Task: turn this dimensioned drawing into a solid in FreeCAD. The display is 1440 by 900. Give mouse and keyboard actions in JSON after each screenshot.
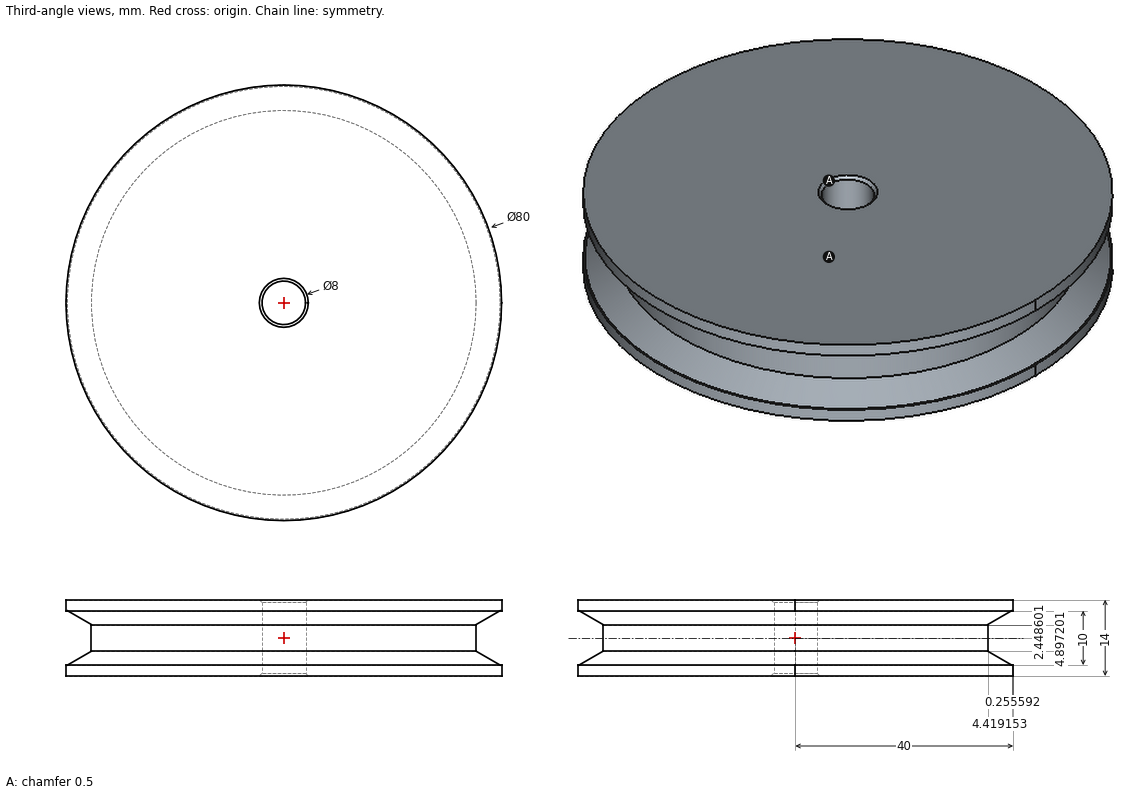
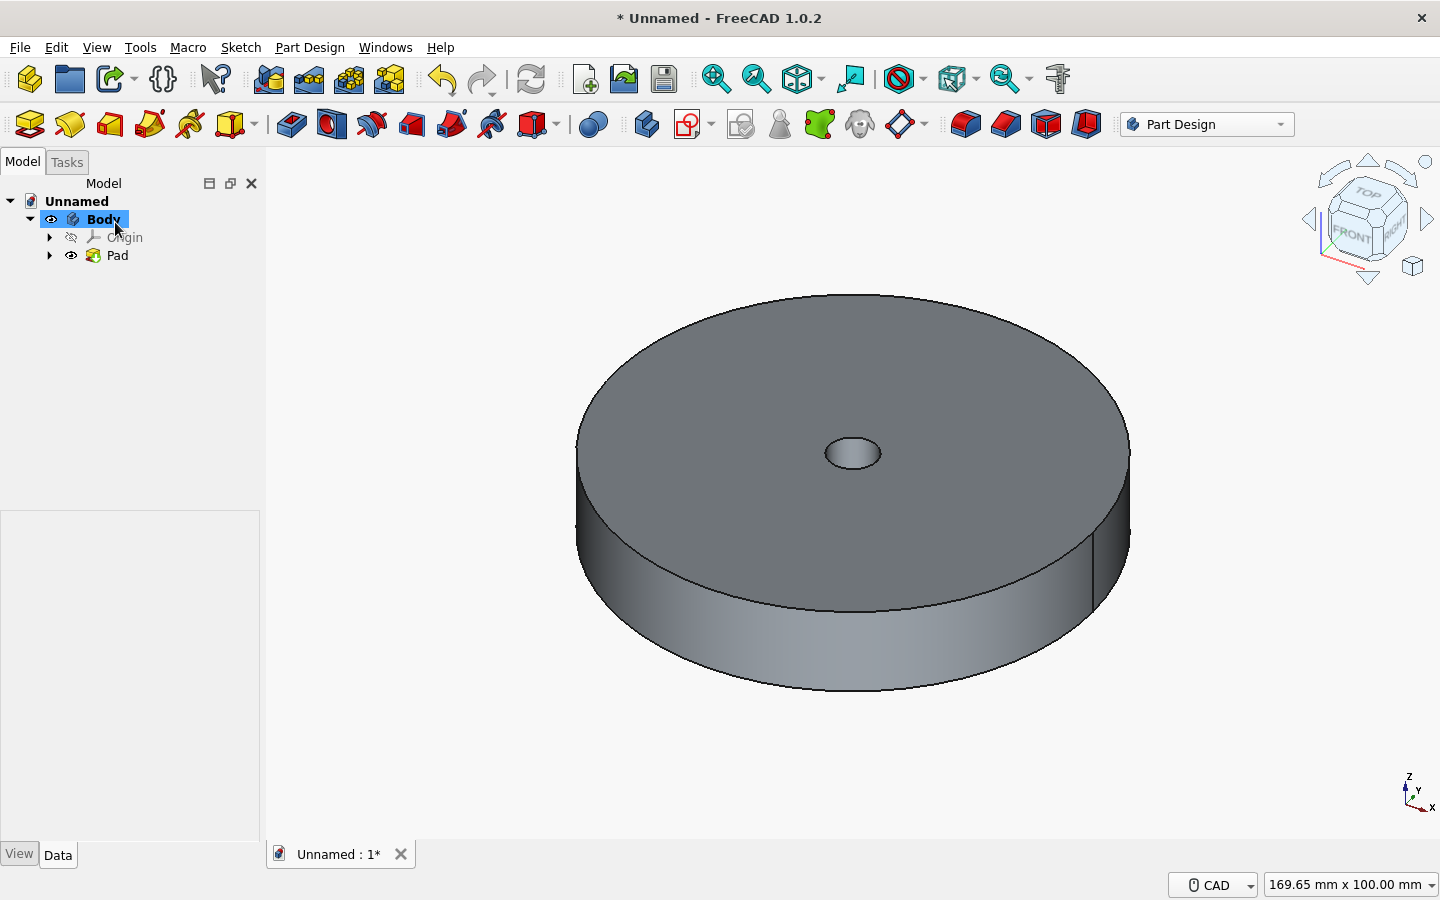
{"action": "left_click", "coordinate": [688, 124]}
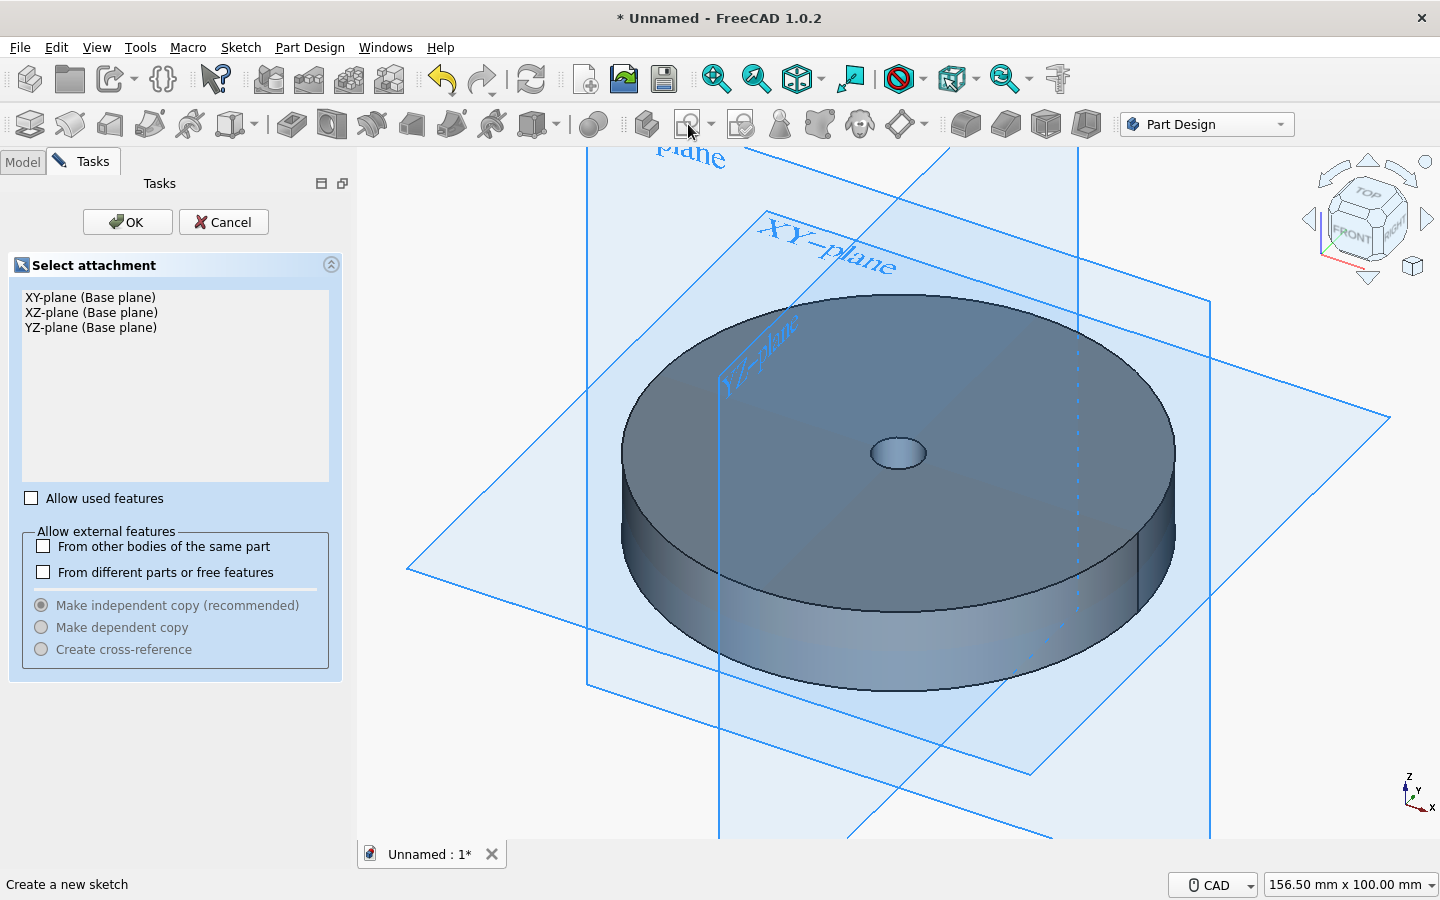
{"action": "left_click", "coordinate": [82, 328]}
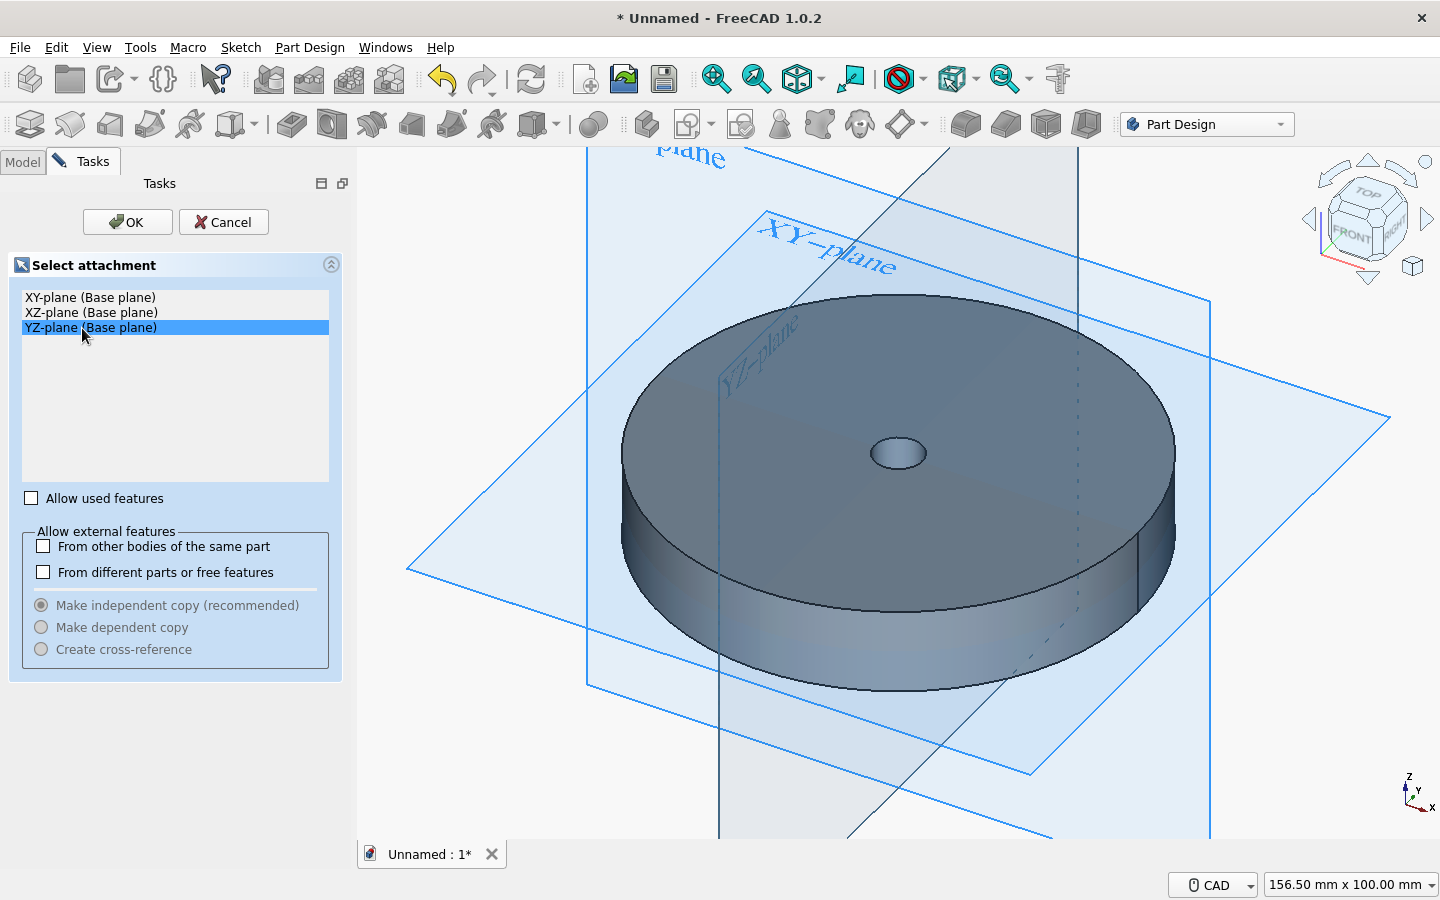
{"action": "left_click", "coordinate": [128, 222]}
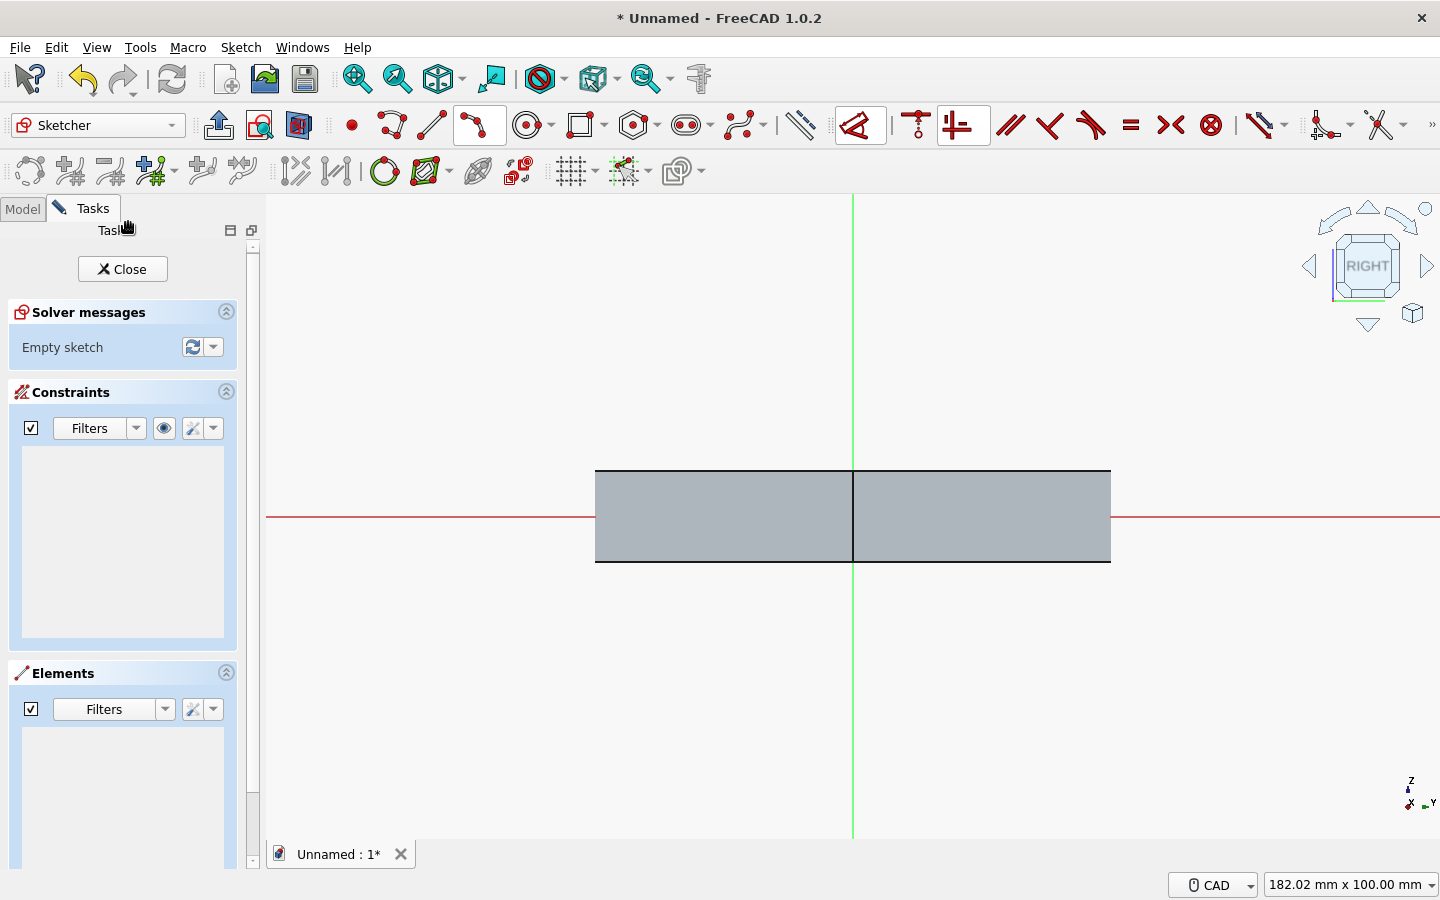
{"action": "left_click", "coordinate": [300, 126]}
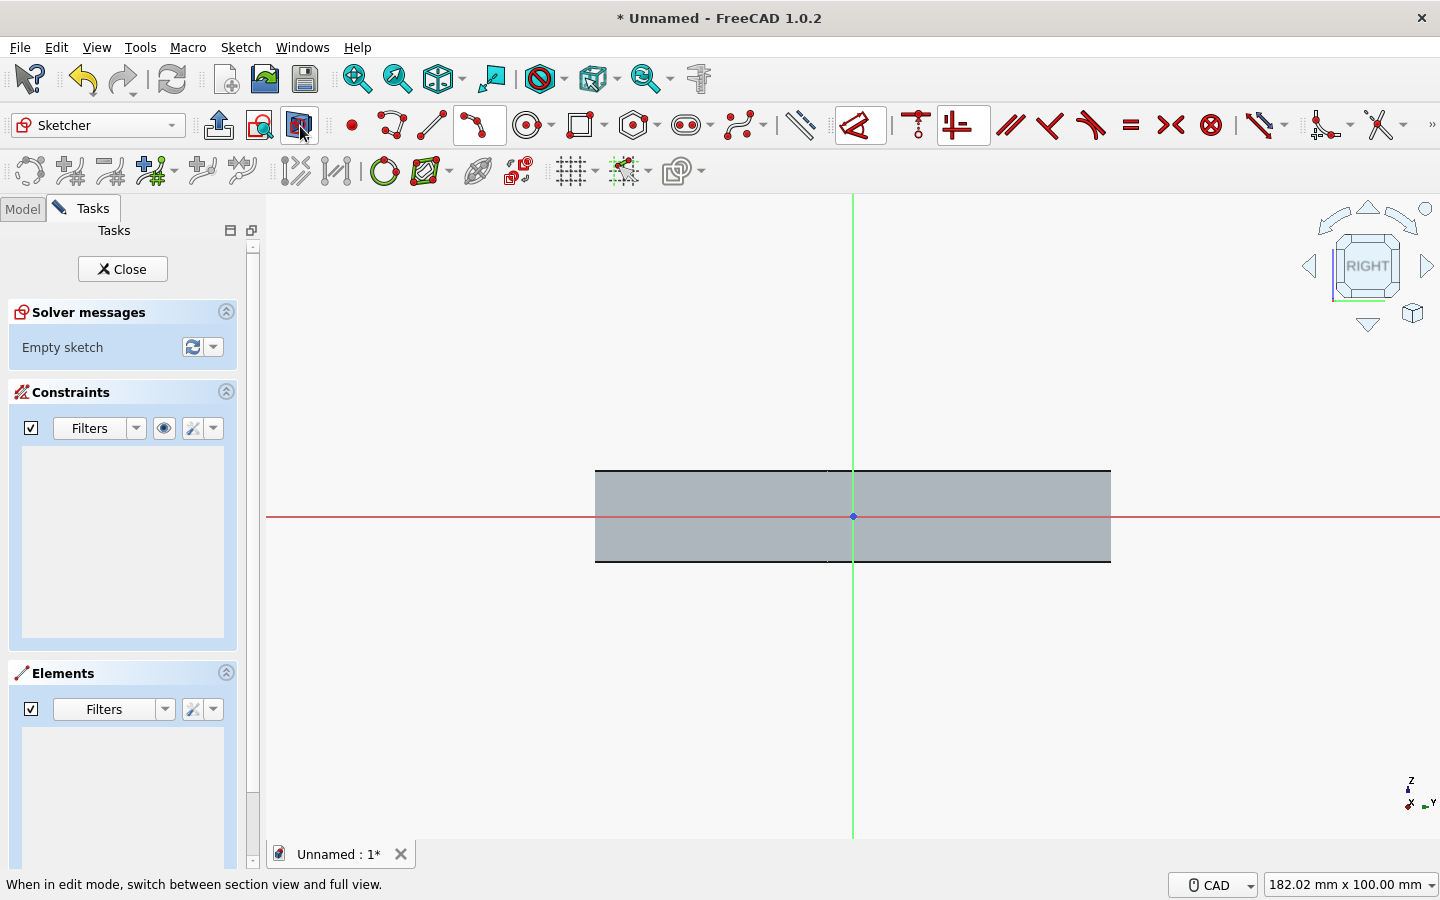
{"action": "scroll", "coordinate": [1158, 516], "scroll_direction": "up", "scroll_amount": 9}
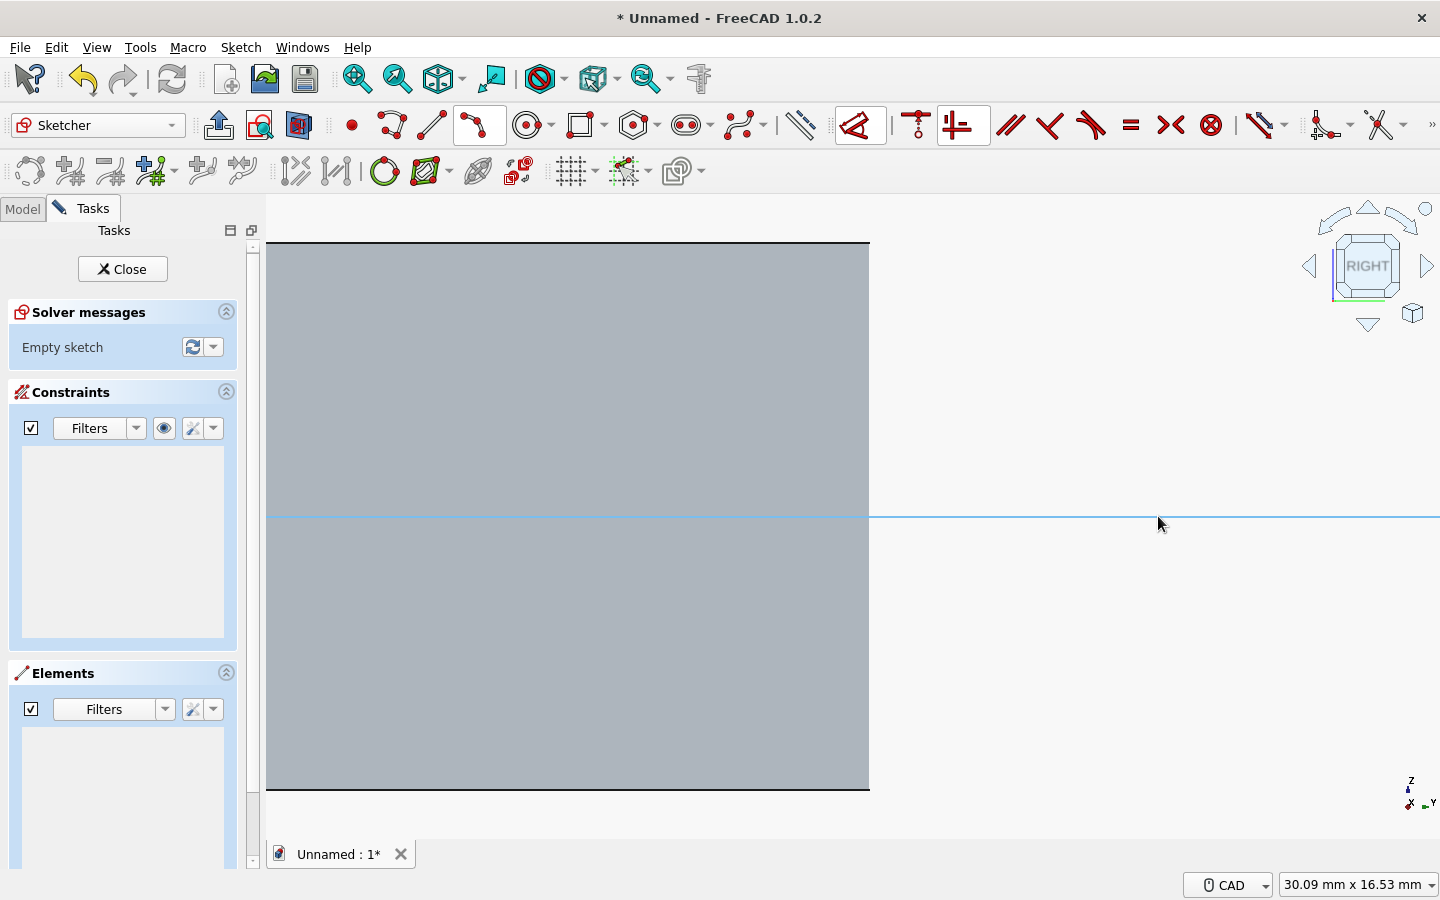
{"action": "left_click", "coordinate": [392, 126]}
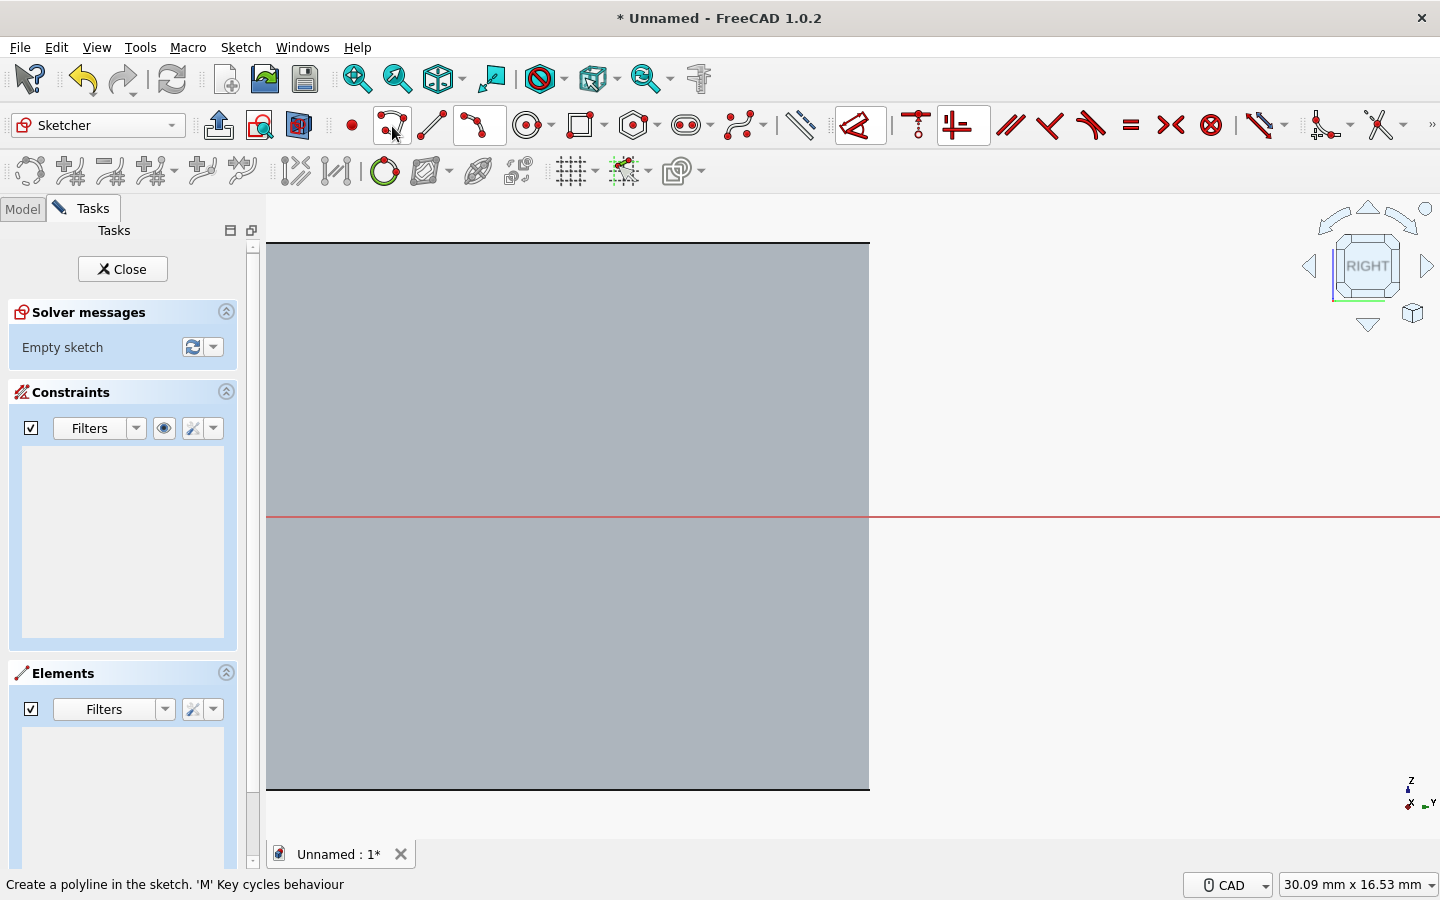
{"action": "left_click", "coordinate": [687, 421]}
{"action": "left_click", "coordinate": [687, 612]}
{"action": "left_click", "coordinate": [860, 712]}